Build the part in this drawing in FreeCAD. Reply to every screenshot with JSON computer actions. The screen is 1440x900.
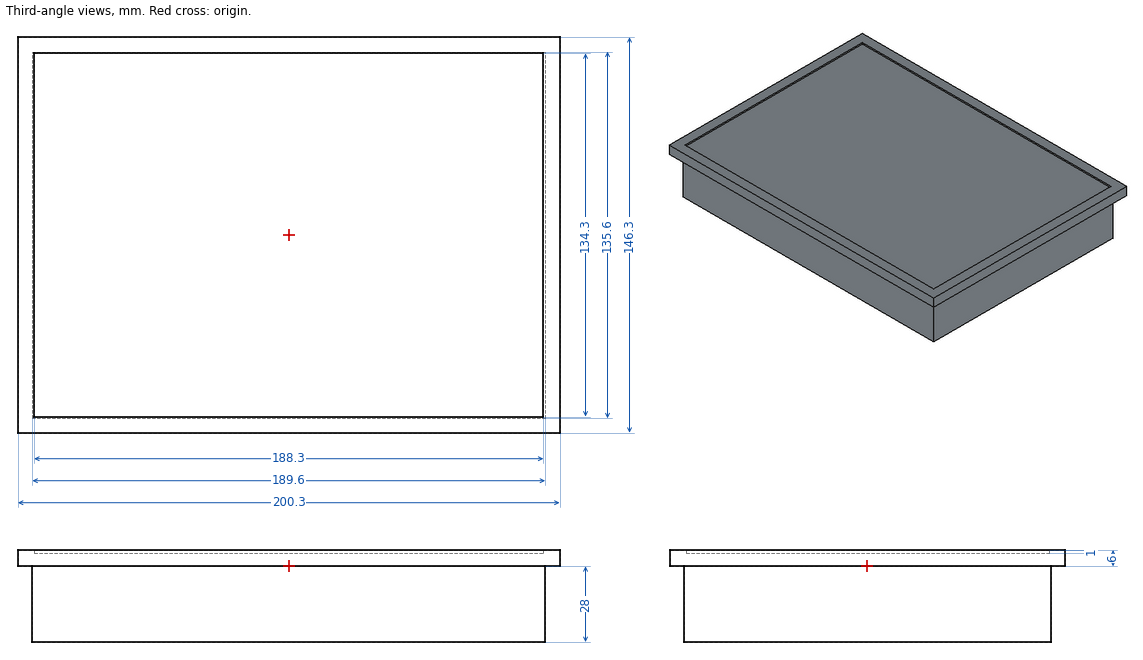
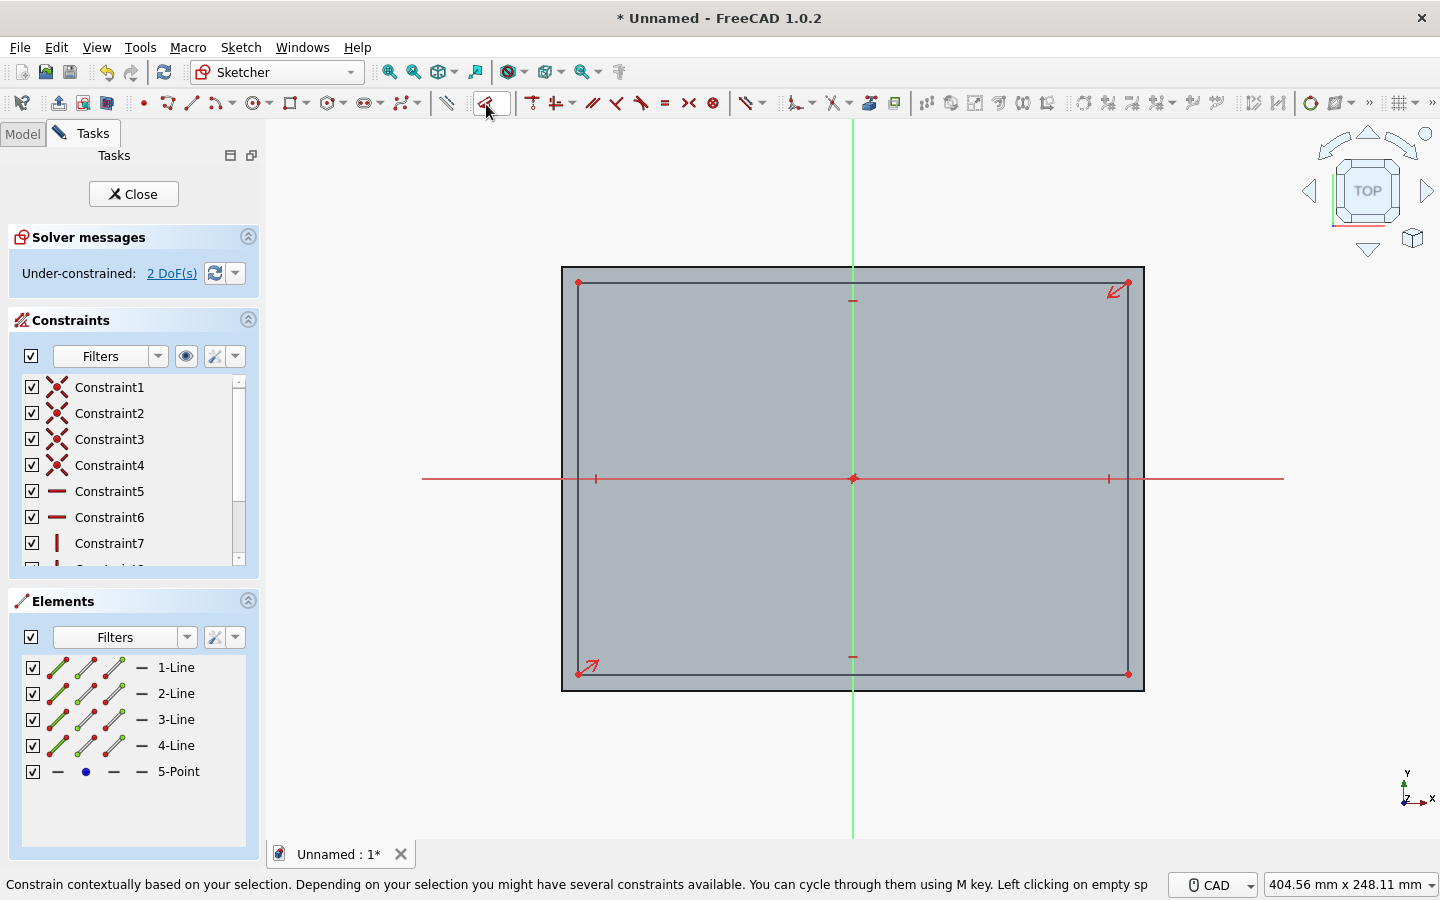
{"action": "left_click", "coordinate": [743, 675]}
{"action": "left_click", "coordinate": [727, 709]}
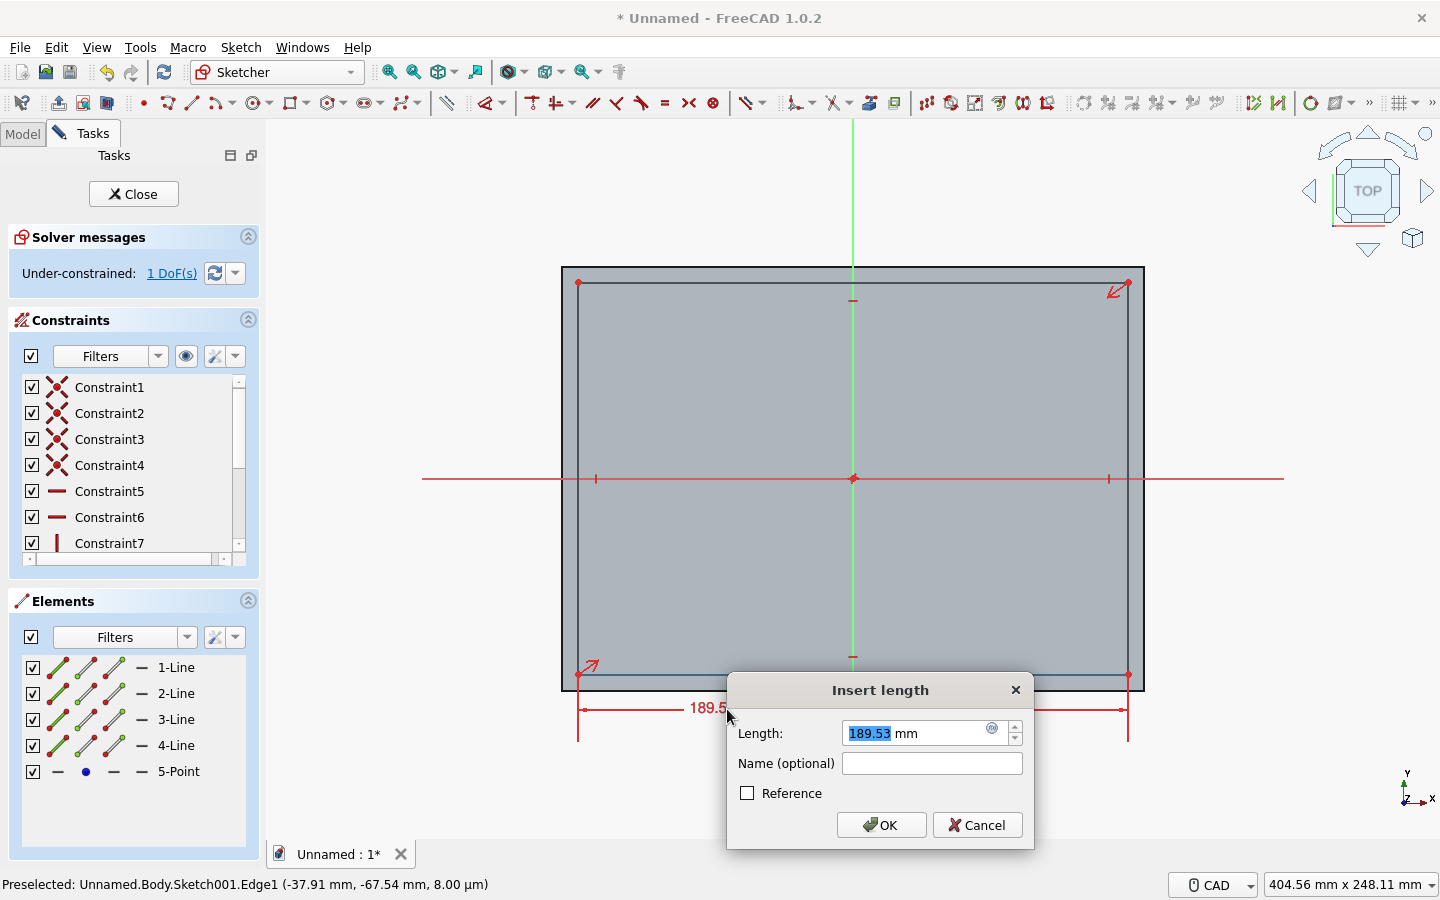
{"action": "type", "text": "189.6"}
{"action": "key", "text": "Return"}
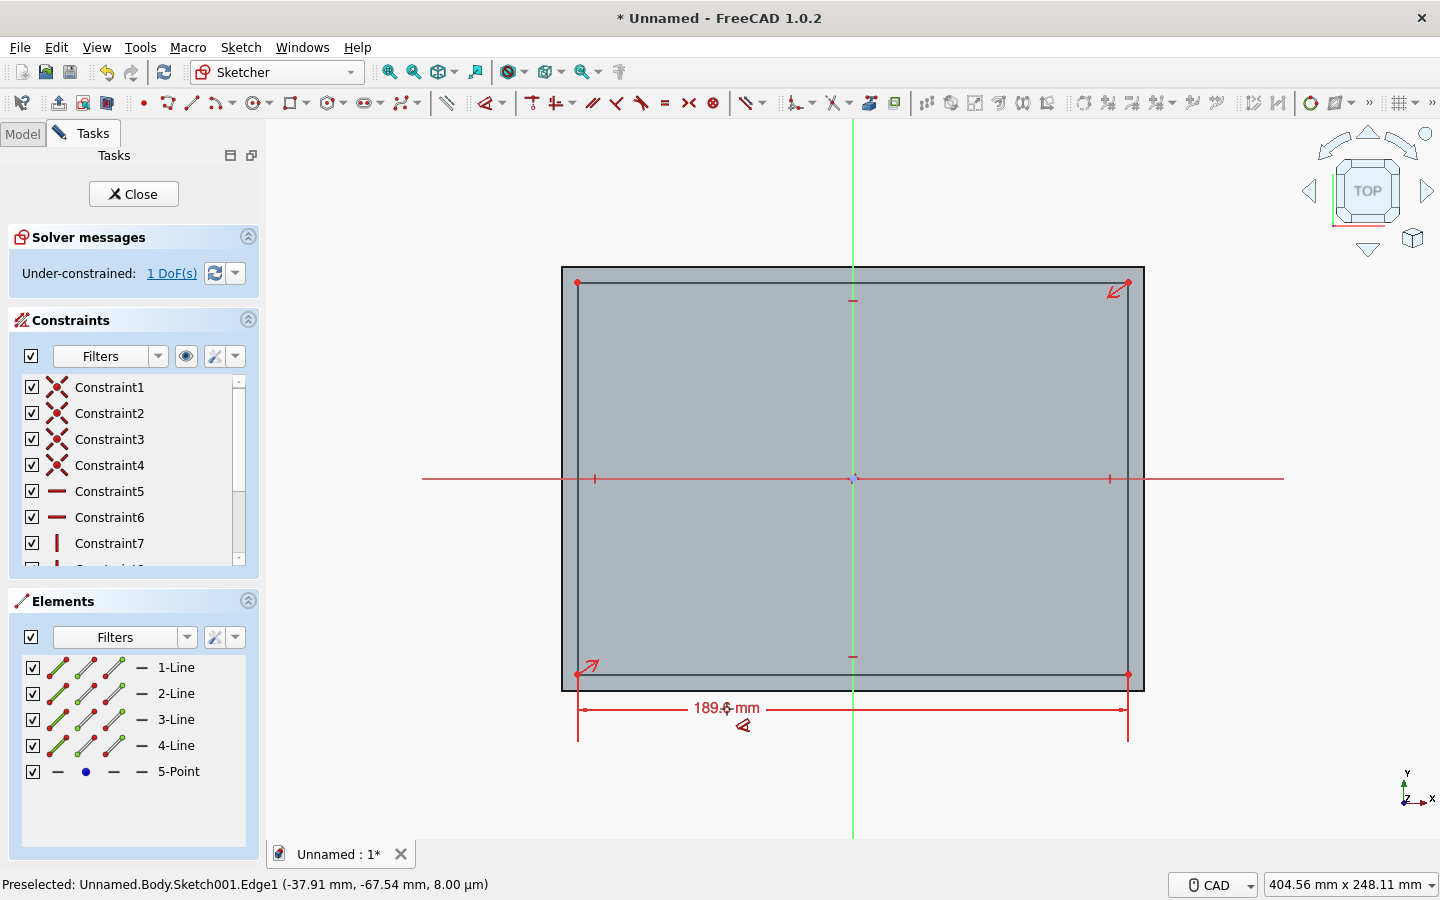
{"action": "left_click", "coordinate": [1128, 557]}
{"action": "left_click", "coordinate": [1162, 389]}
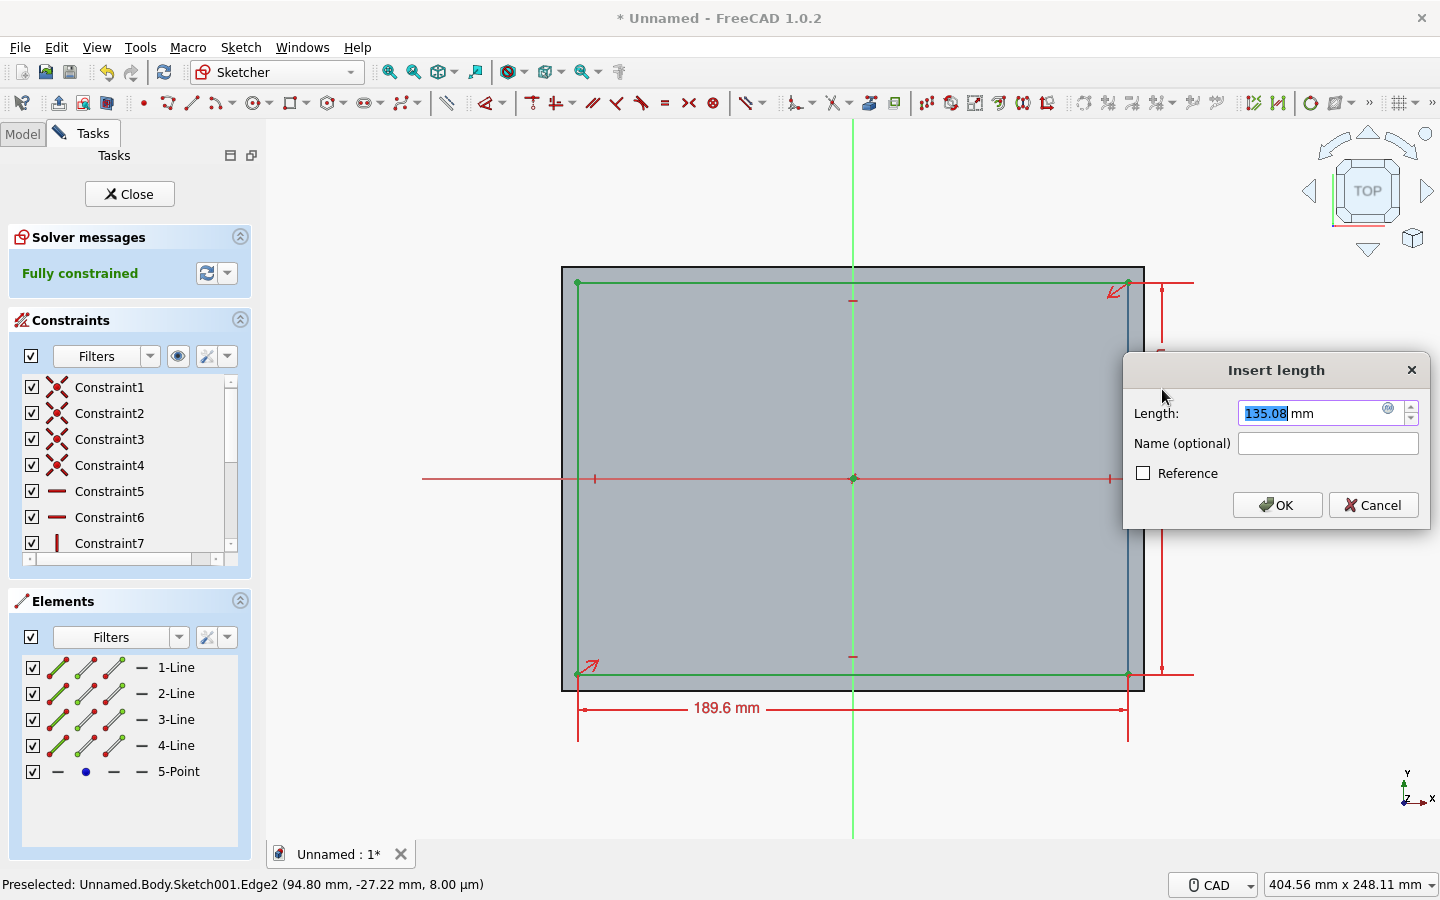
{"action": "type", "text": "135.6"}
{"action": "key", "text": "Return"}
{"action": "key", "text": "Escape"}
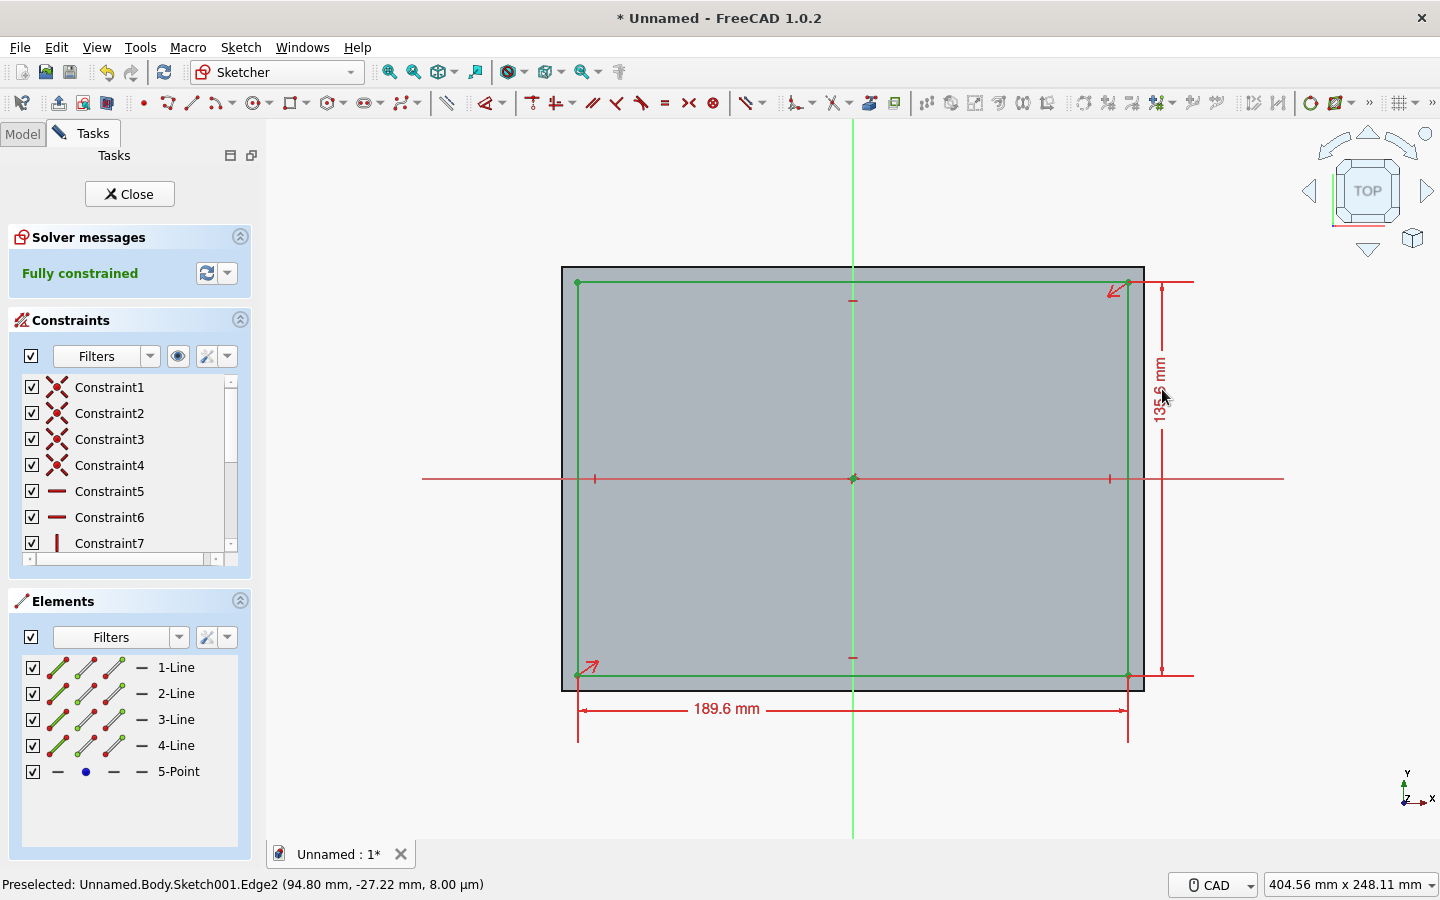
{"action": "left_click", "coordinate": [130, 194]}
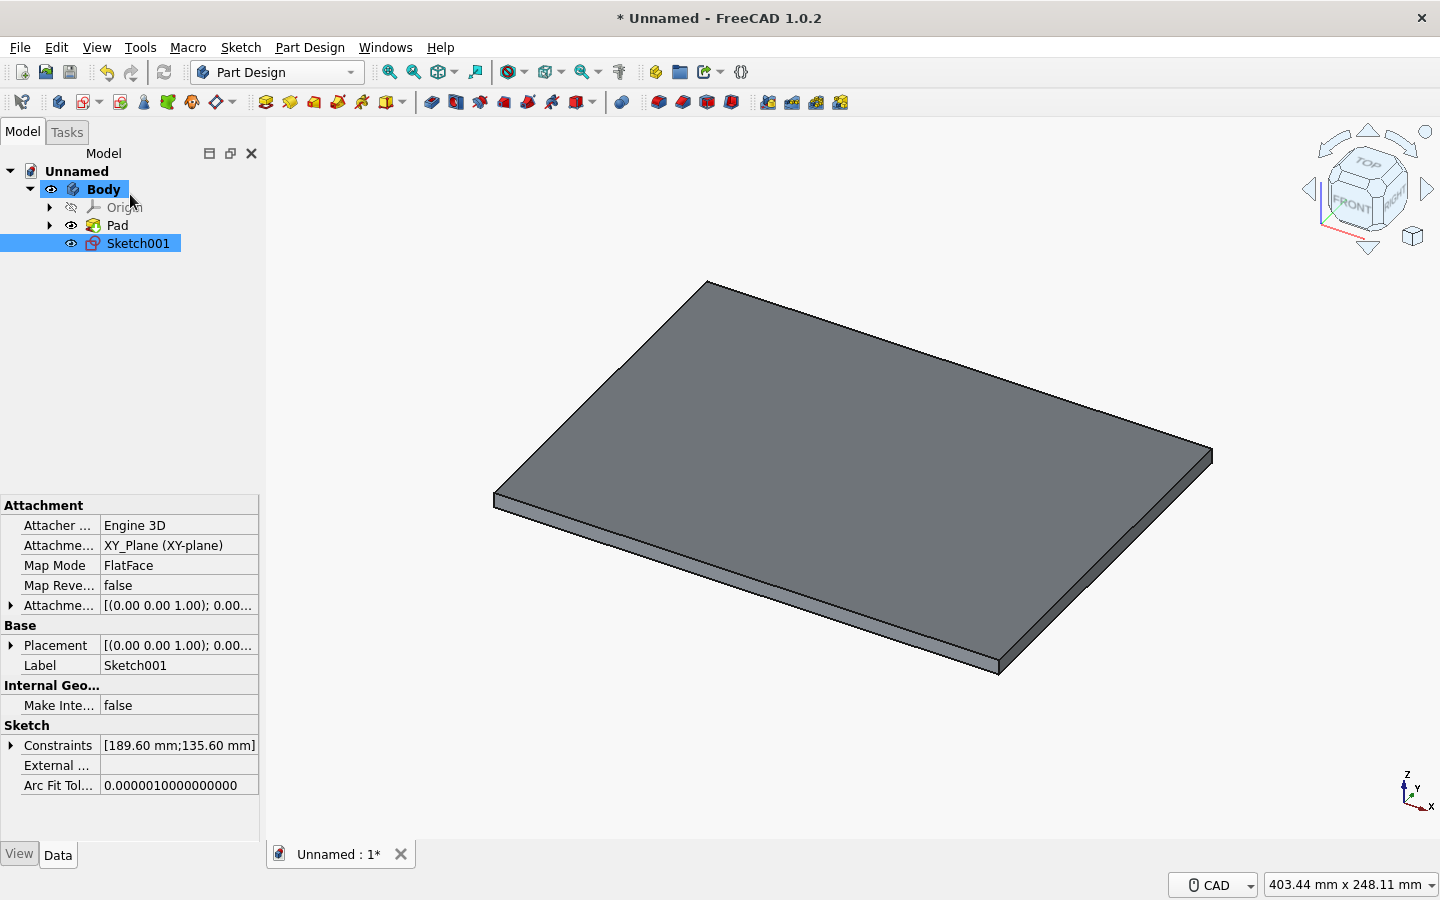
{"action": "left_click", "coordinate": [266, 102]}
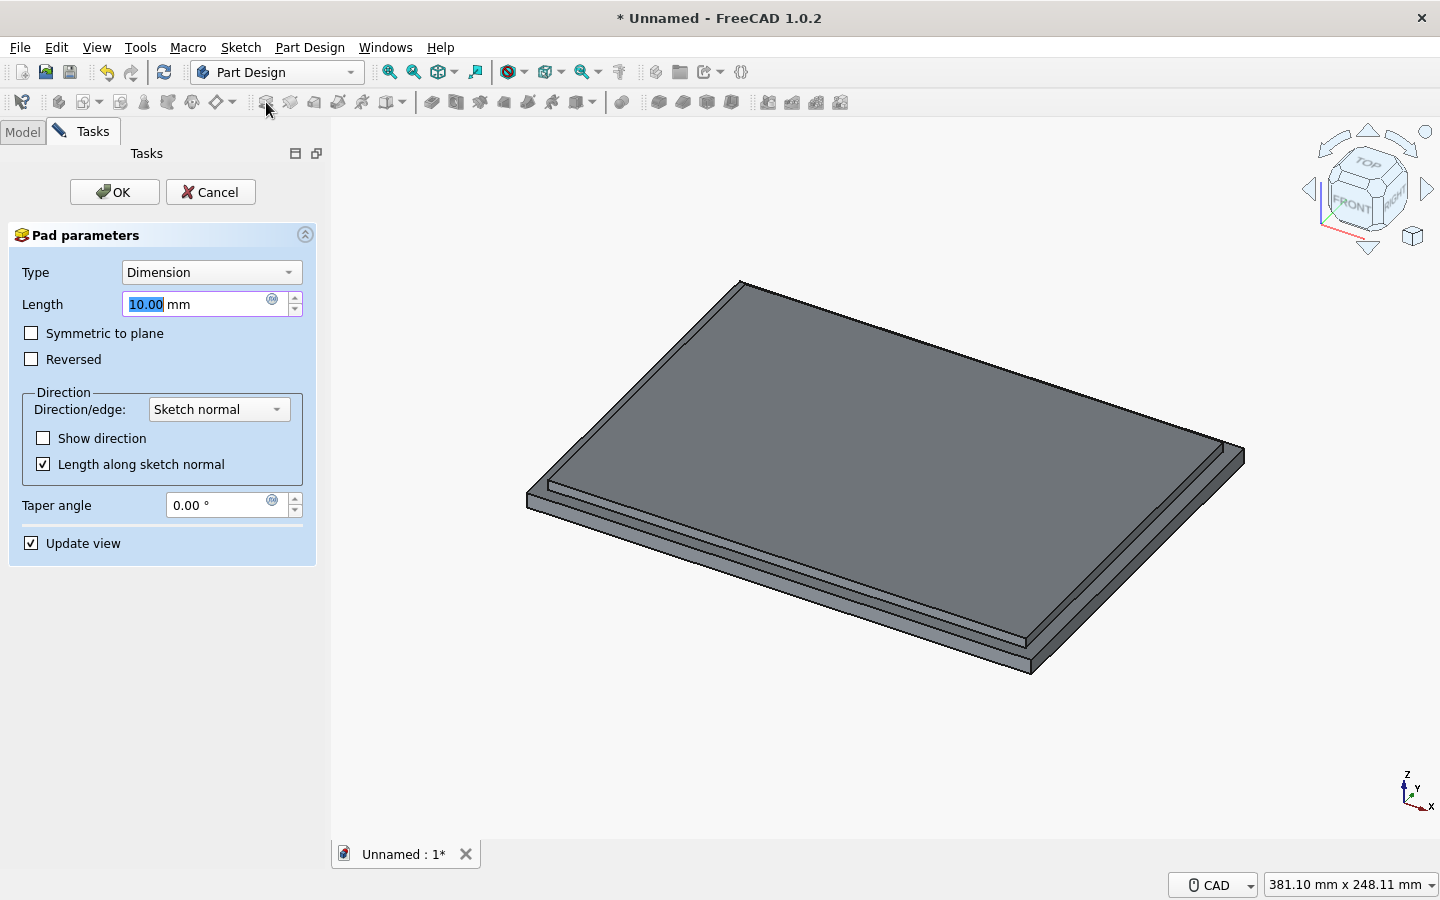
{"action": "type", "text": "28"}
{"action": "key", "text": "Tab"}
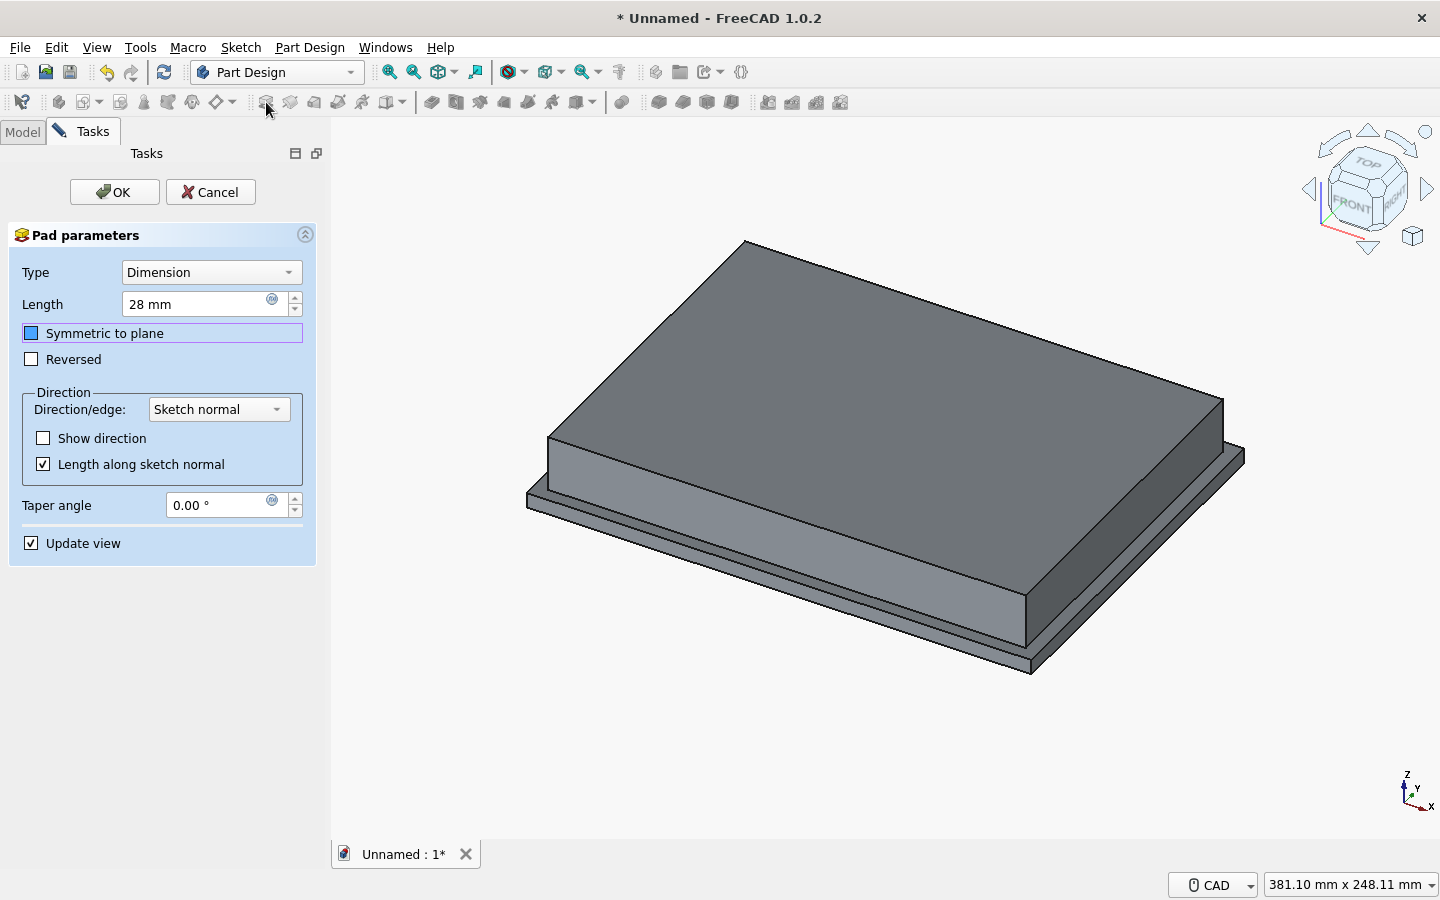
{"action": "left_click", "coordinate": [30, 359]}